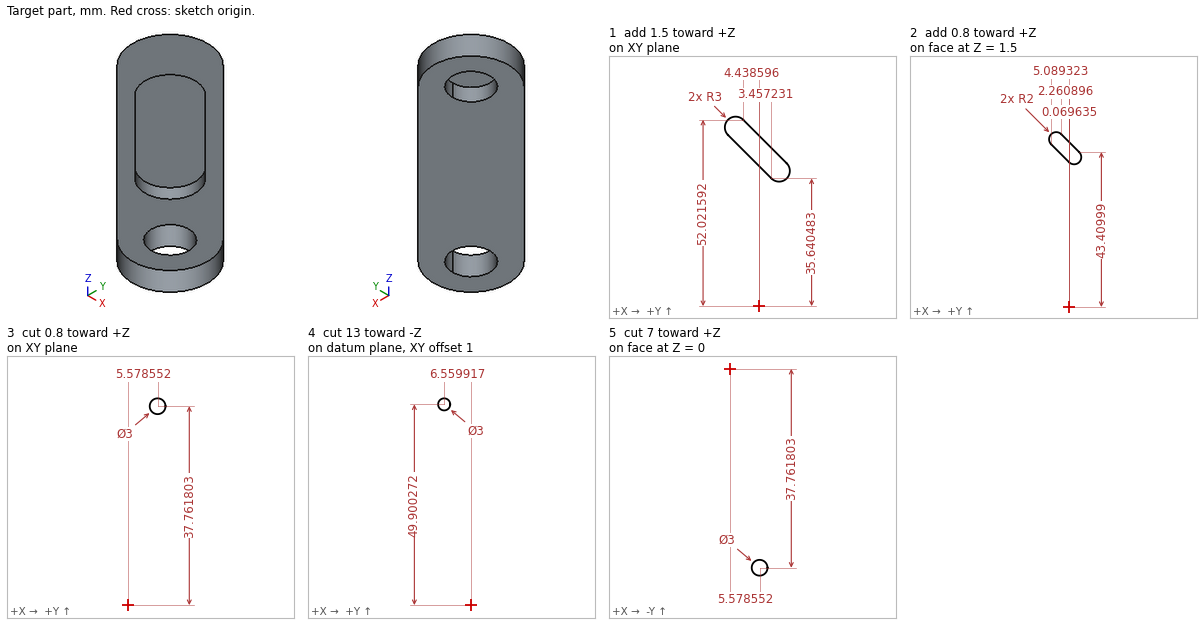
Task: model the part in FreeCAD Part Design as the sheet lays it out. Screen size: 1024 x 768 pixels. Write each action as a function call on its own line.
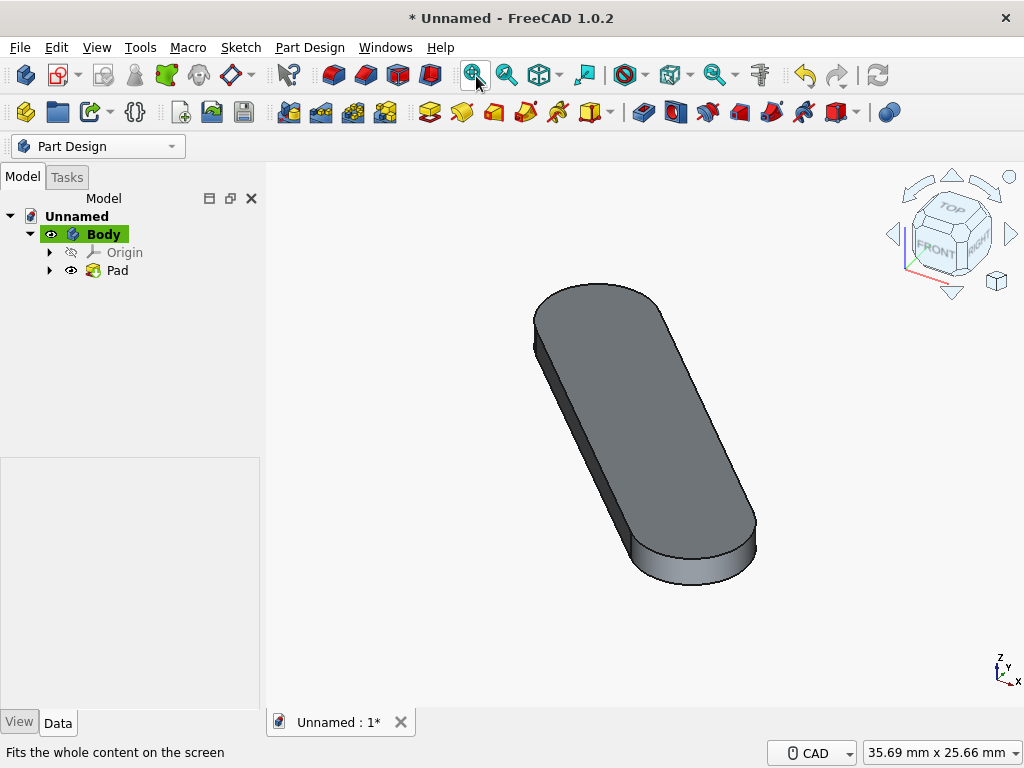
click(645, 420)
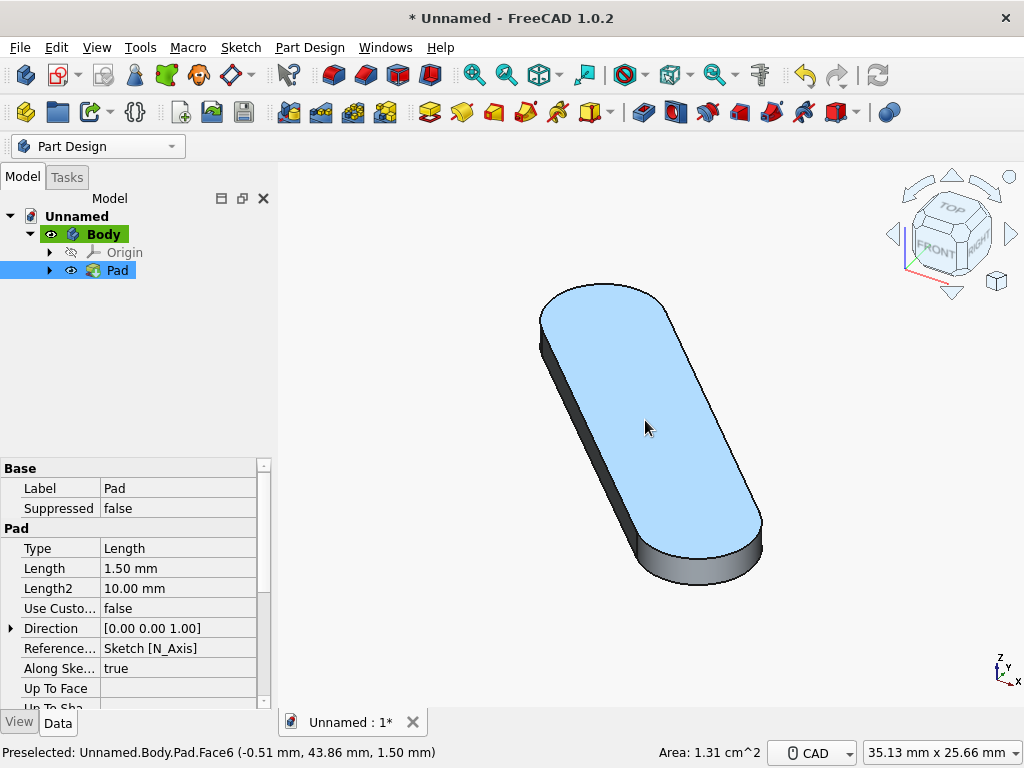
click(58, 76)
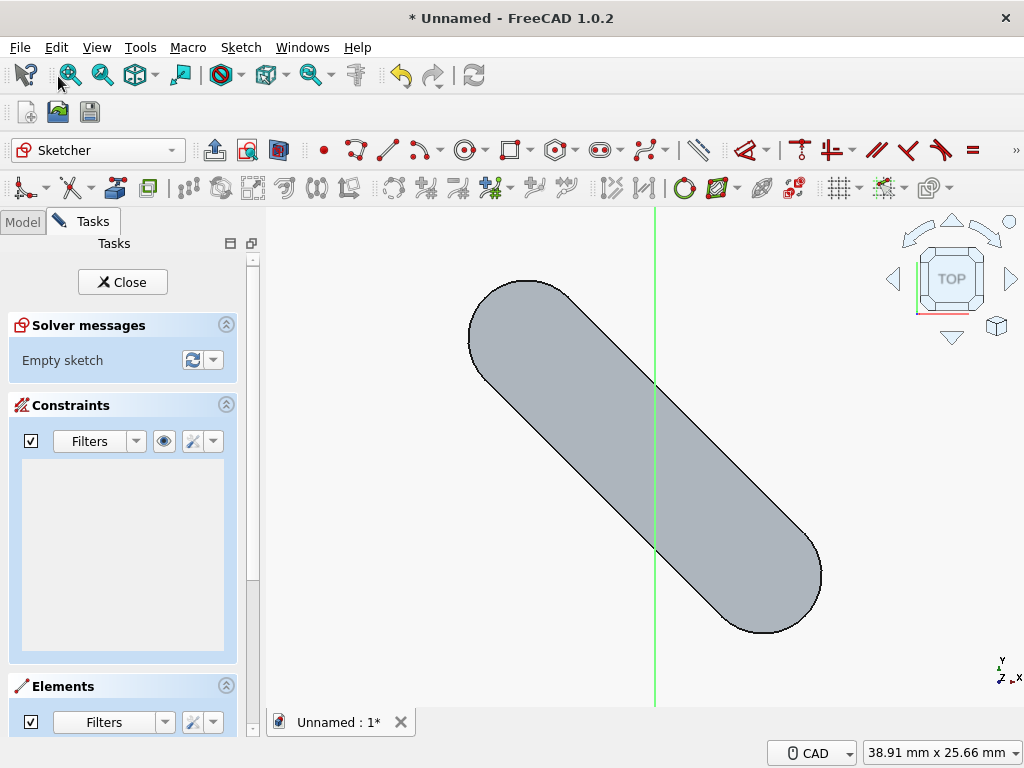
scroll(677, 433, up, 4)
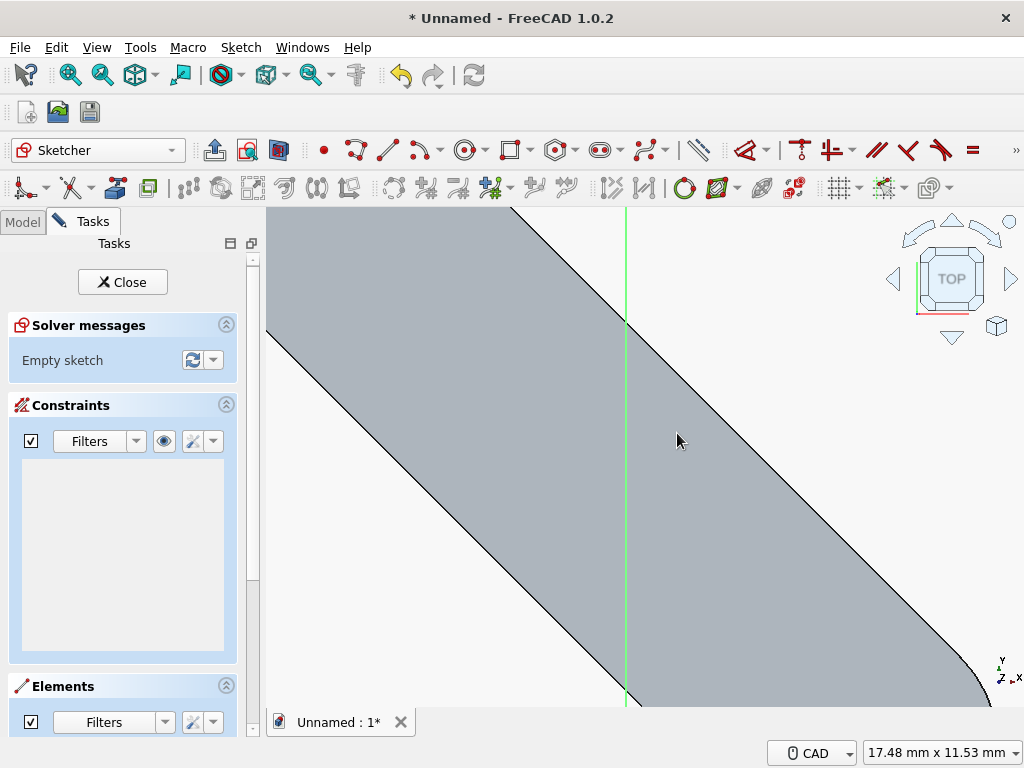
click(600, 150)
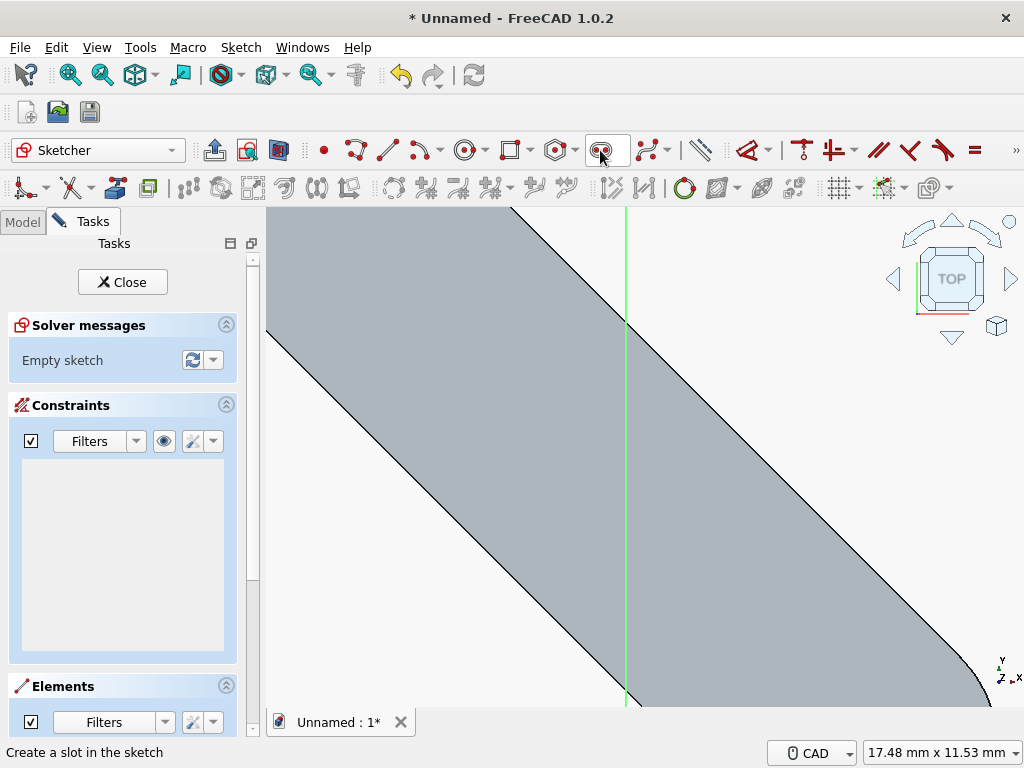
click(467, 348)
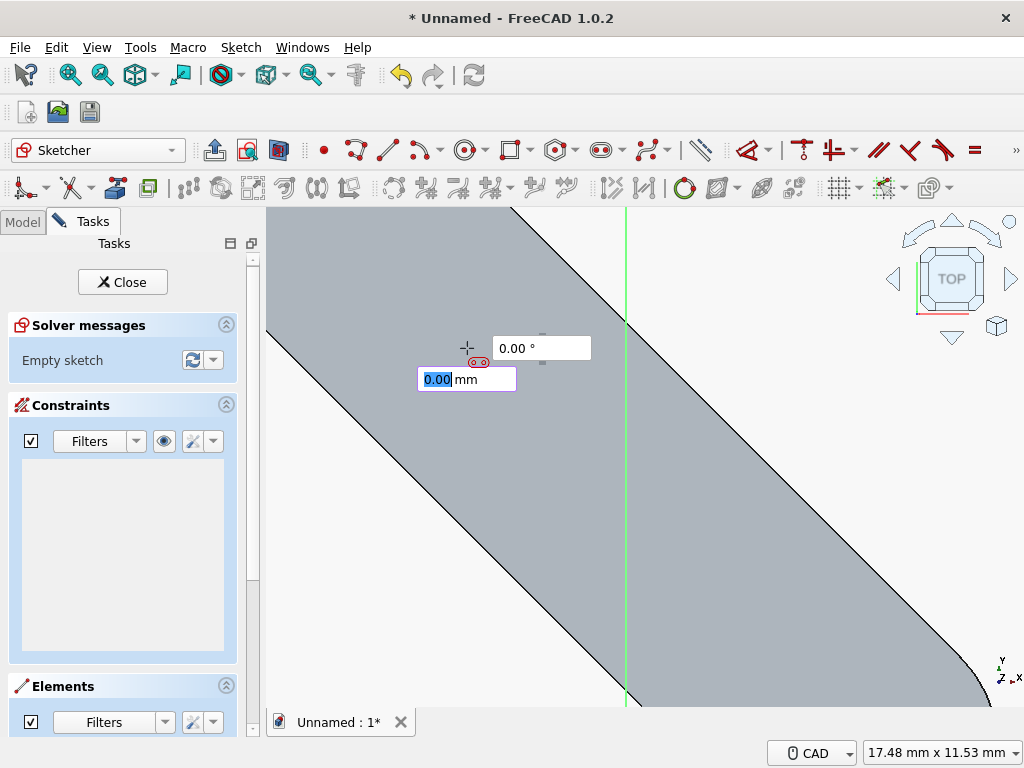
click(685, 565)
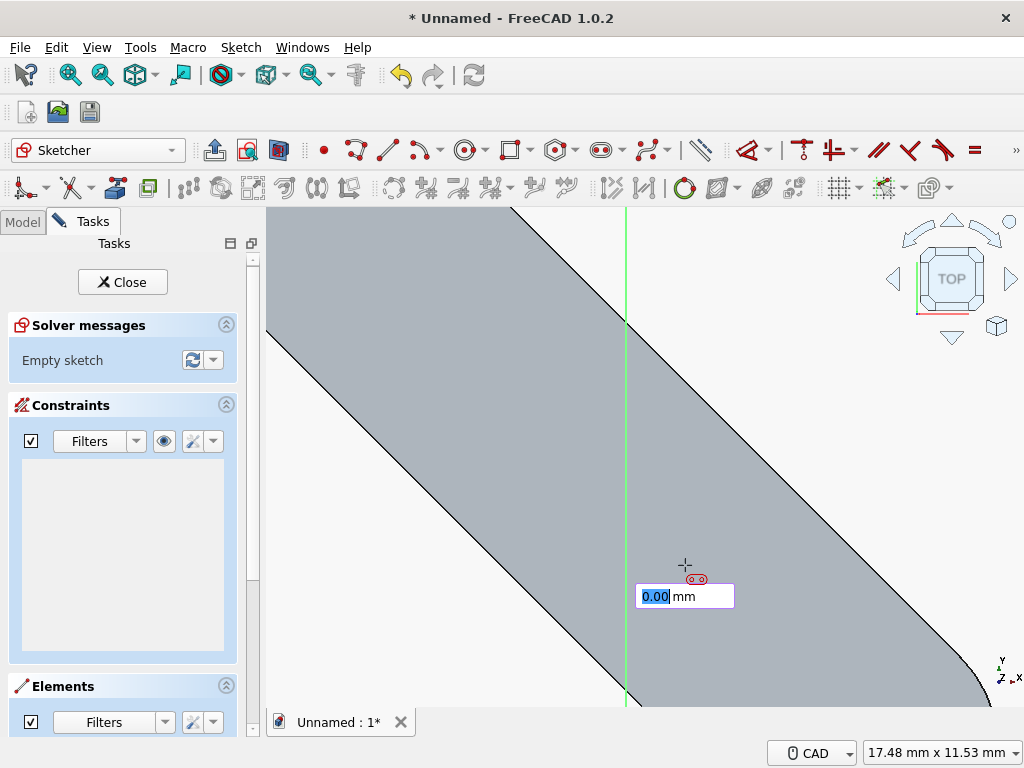
click(670, 428)
key(Escape)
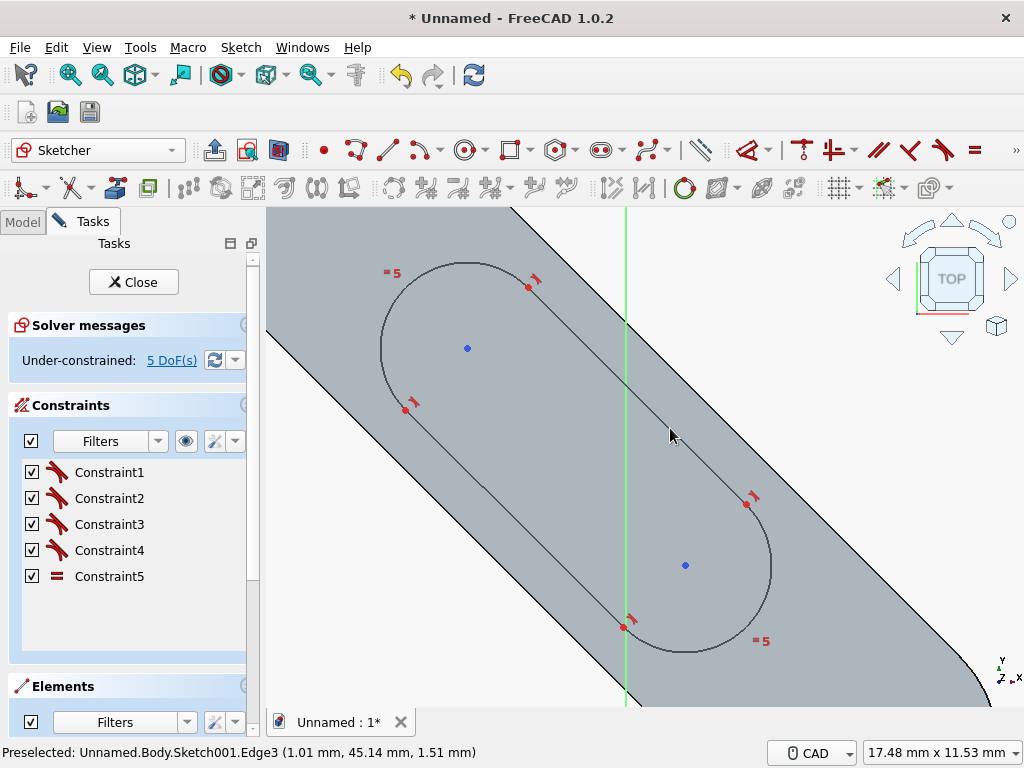
click(748, 150)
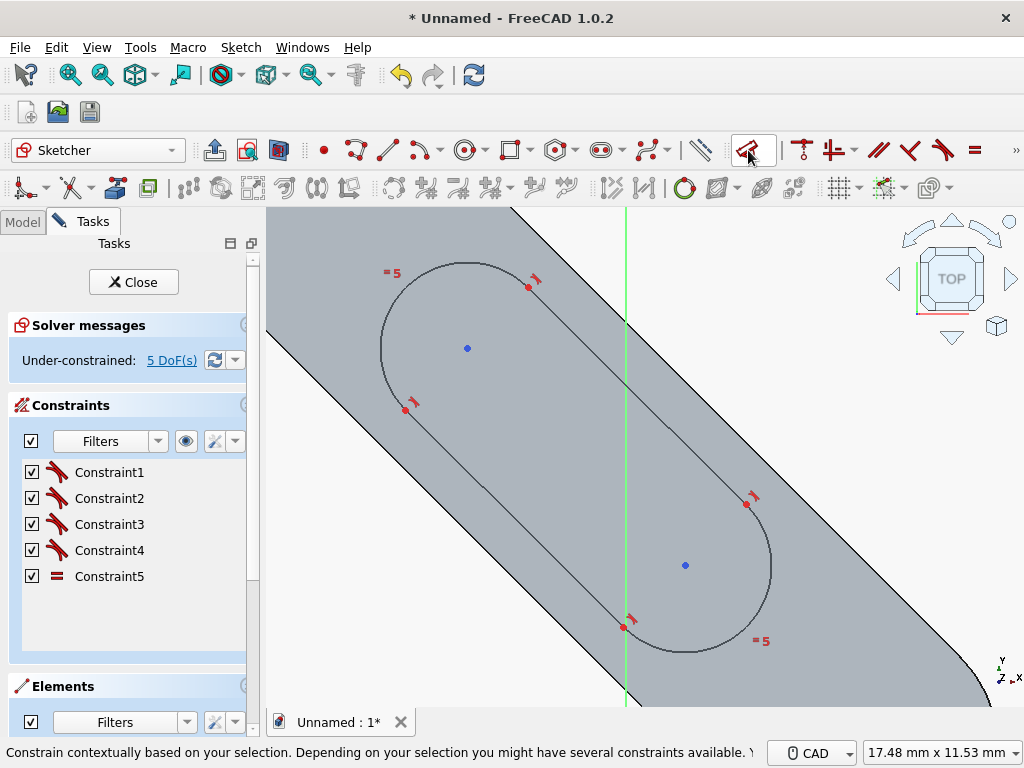
click(453, 264)
click(506, 237)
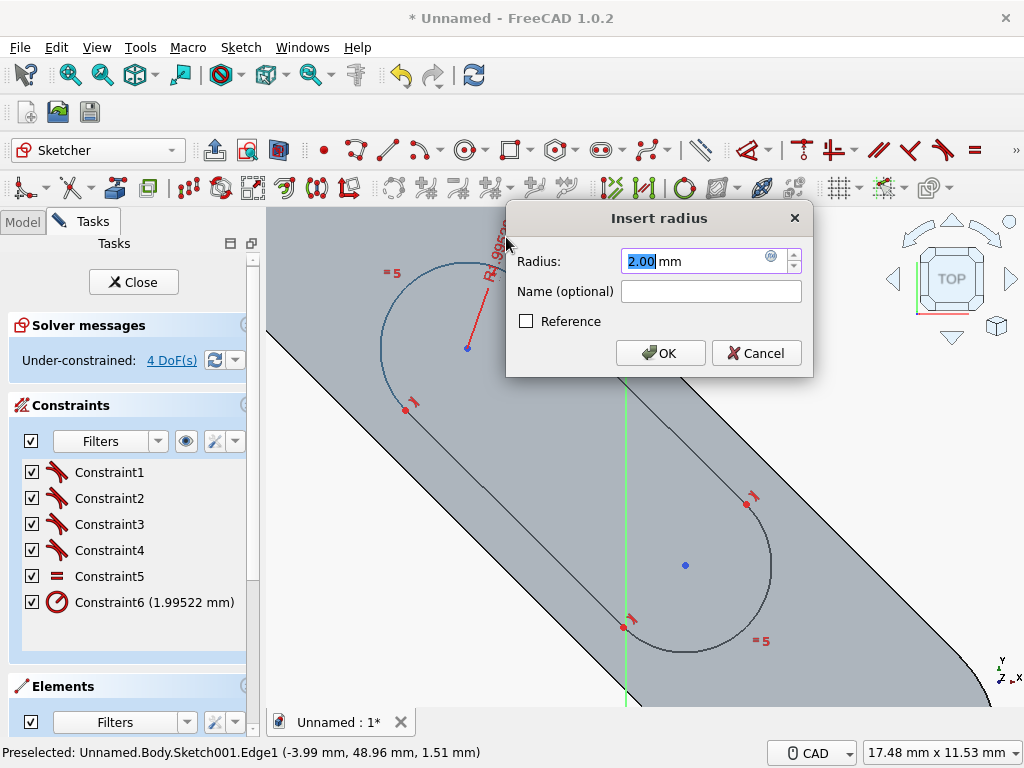
text(2)
key(Return)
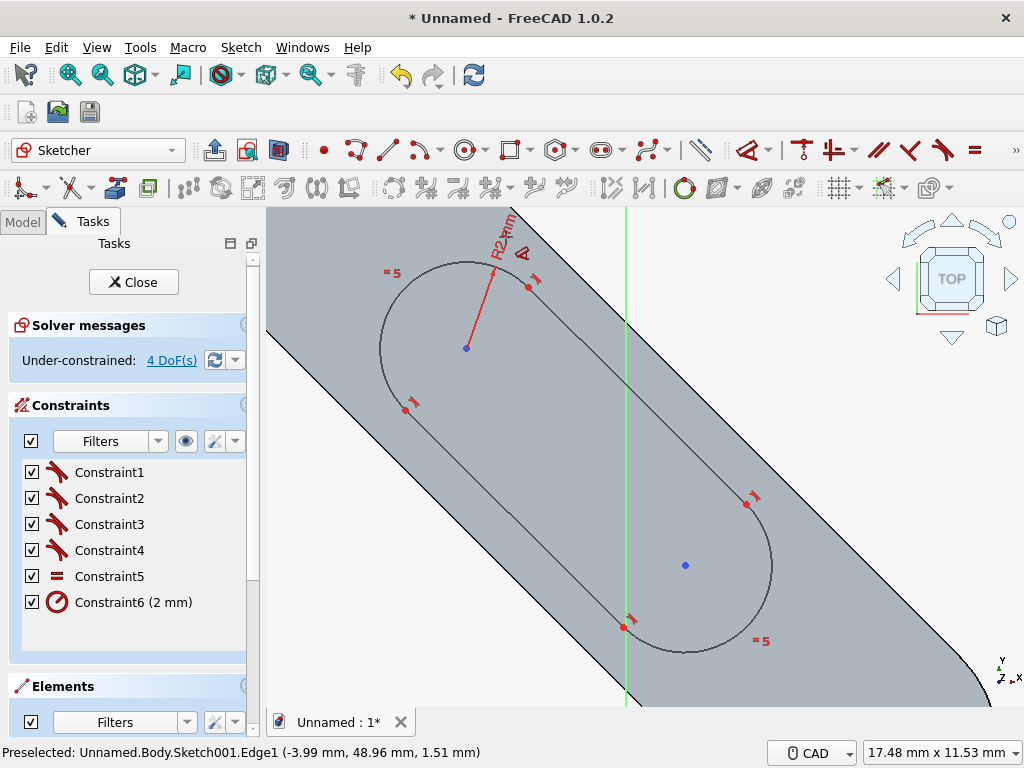
click(528, 287)
click(577, 253)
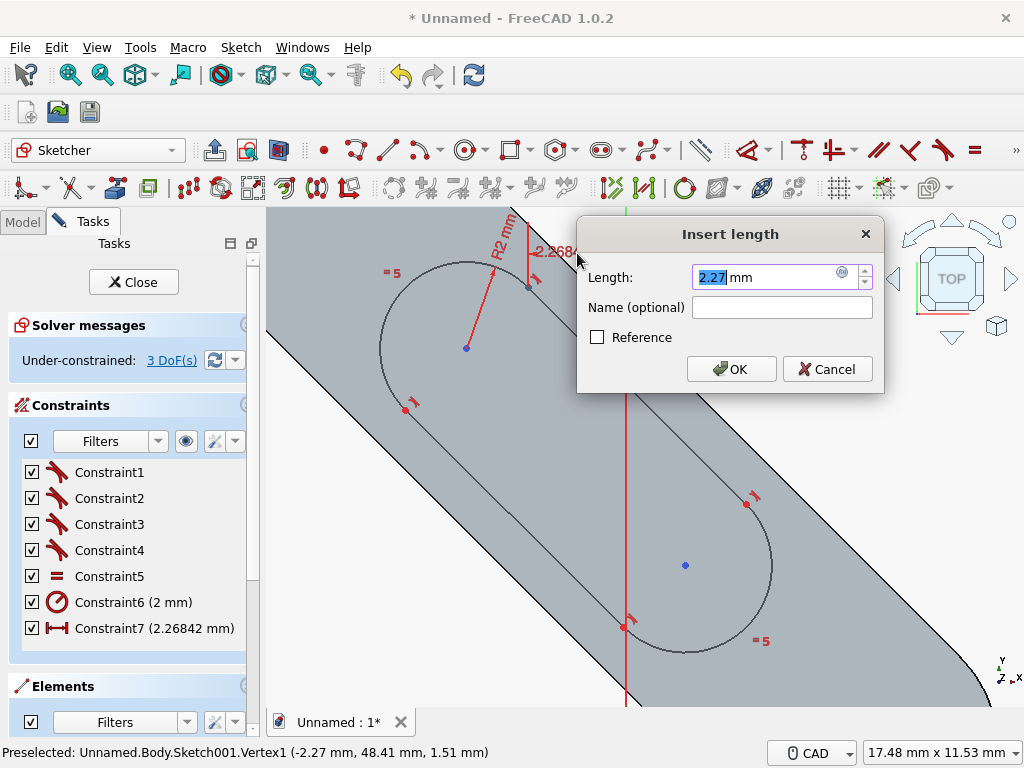
text(2.260896)
key(Return)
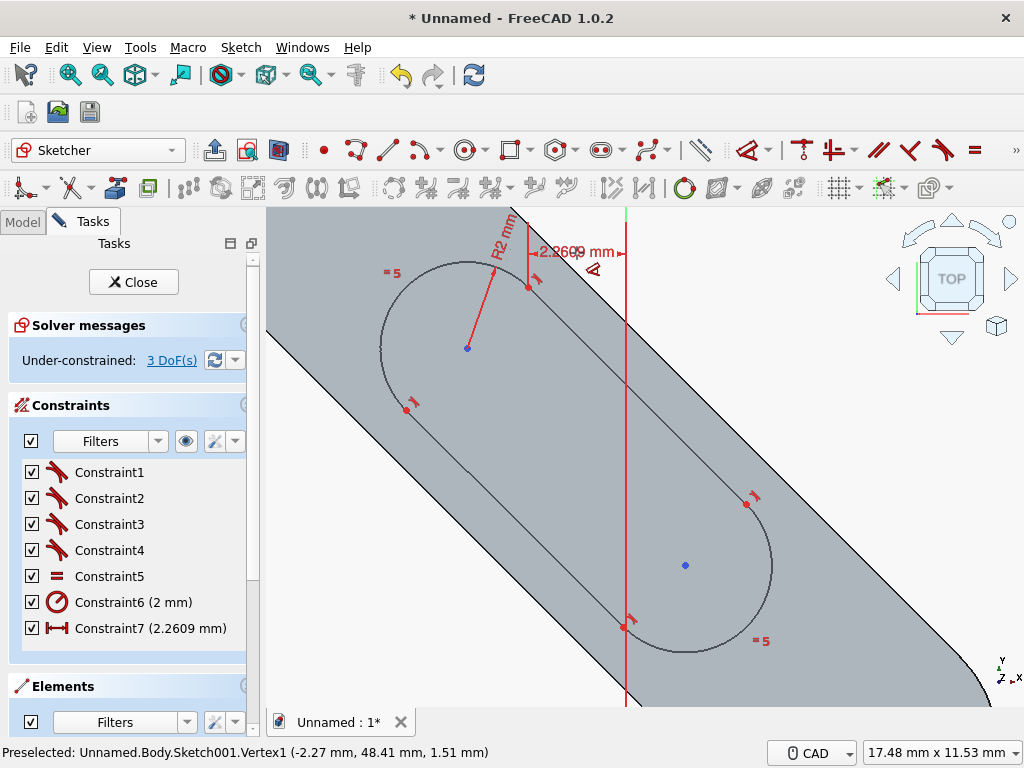
click(406, 410)
click(516, 376)